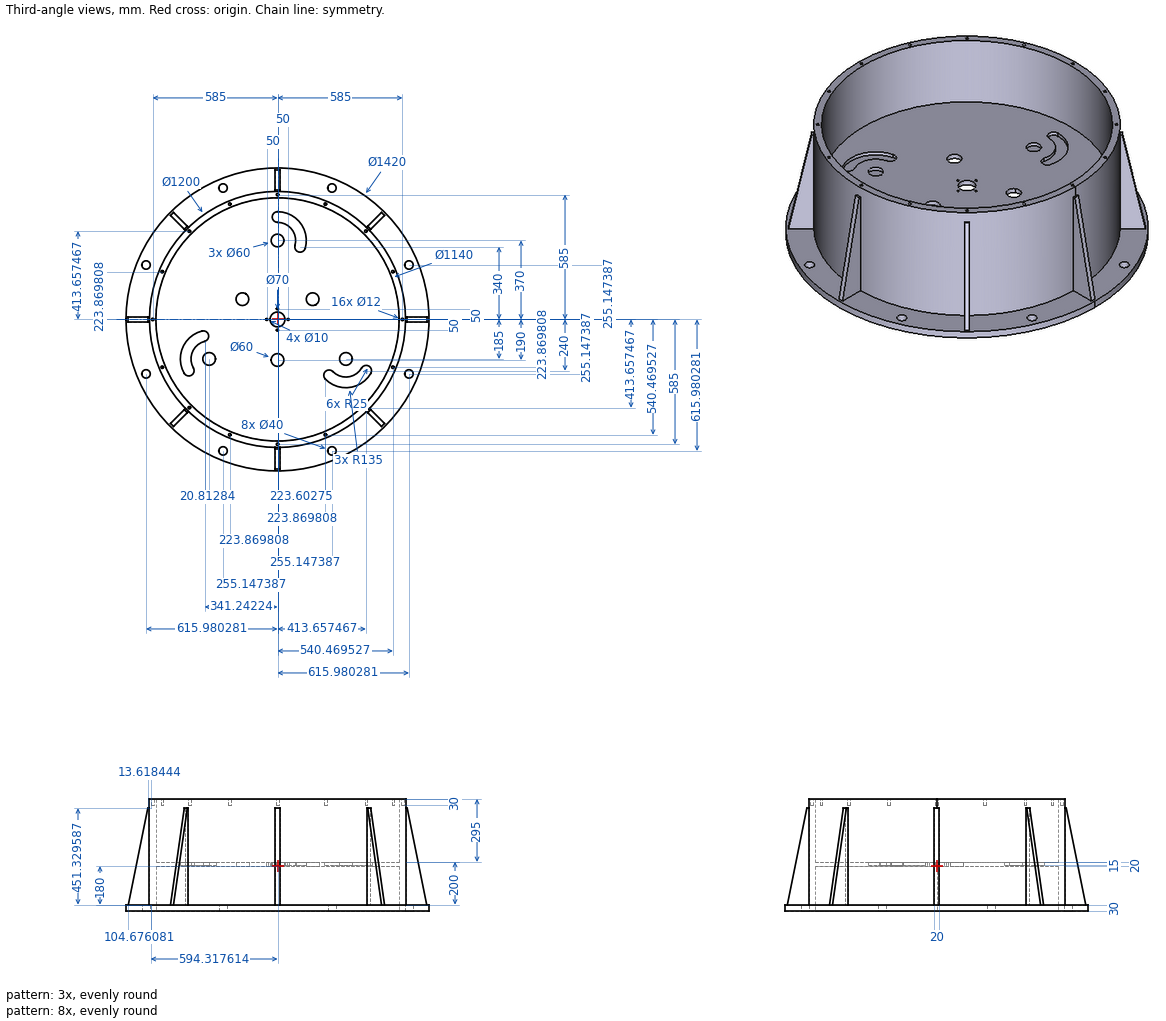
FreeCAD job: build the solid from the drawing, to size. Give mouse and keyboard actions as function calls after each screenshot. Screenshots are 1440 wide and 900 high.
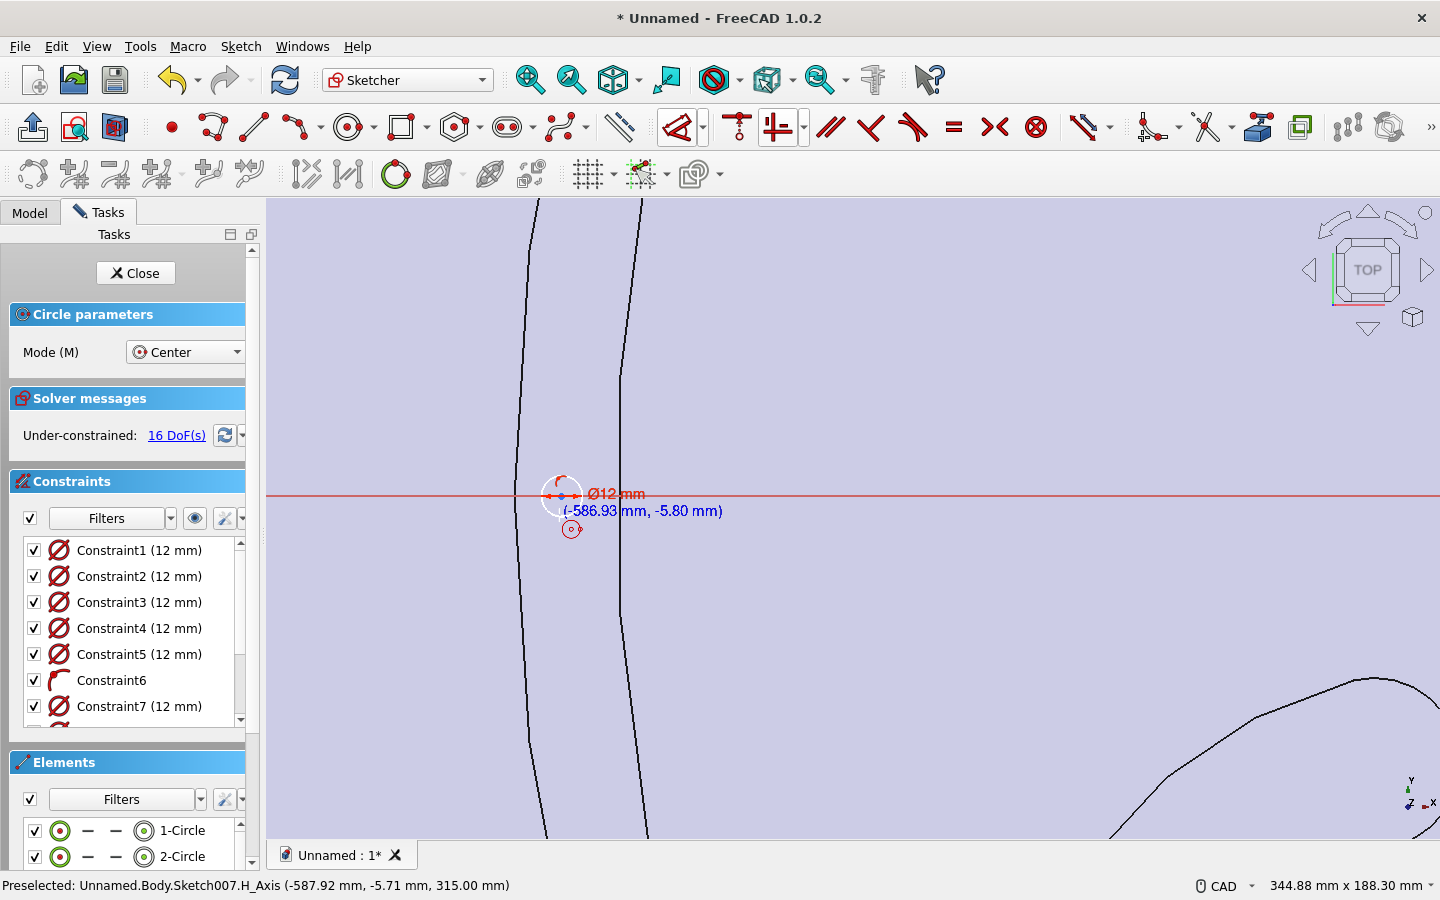
scroll(564, 521, down, 11)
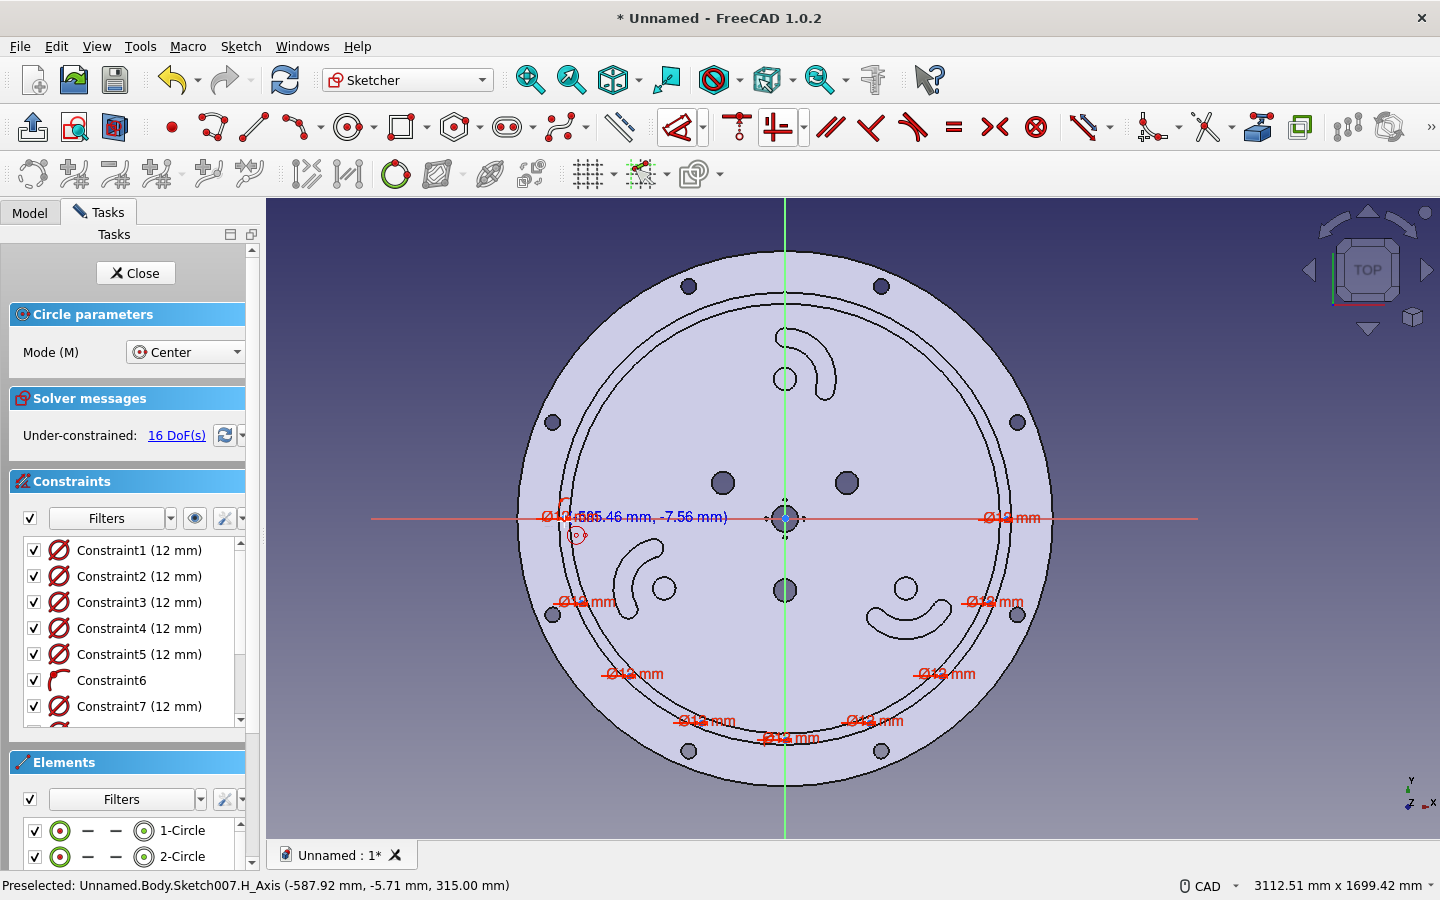
scroll(581, 434, up, 12)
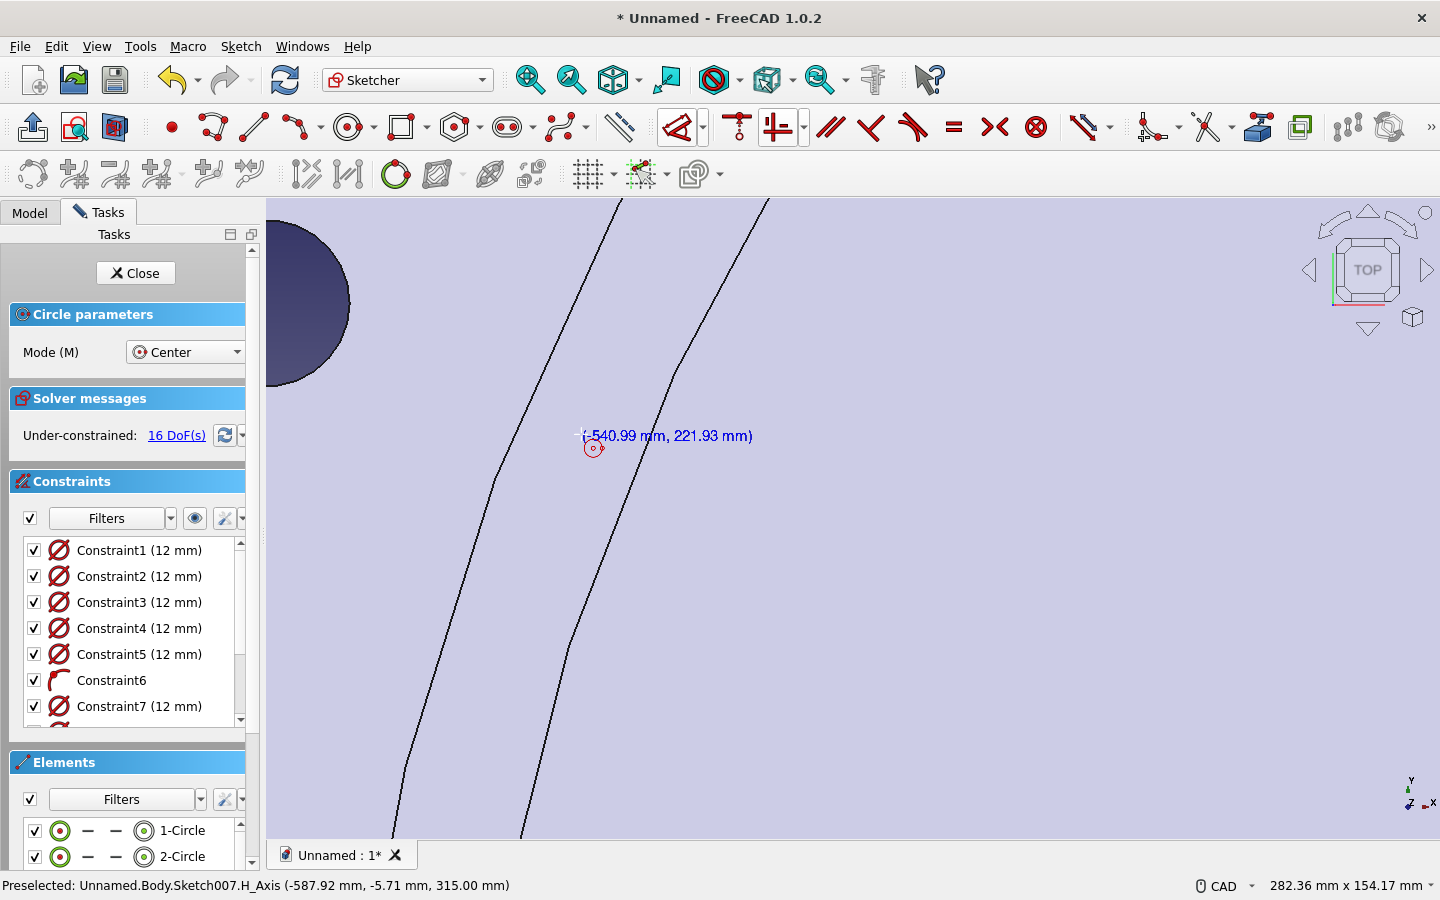
scroll(581, 434, down, 12)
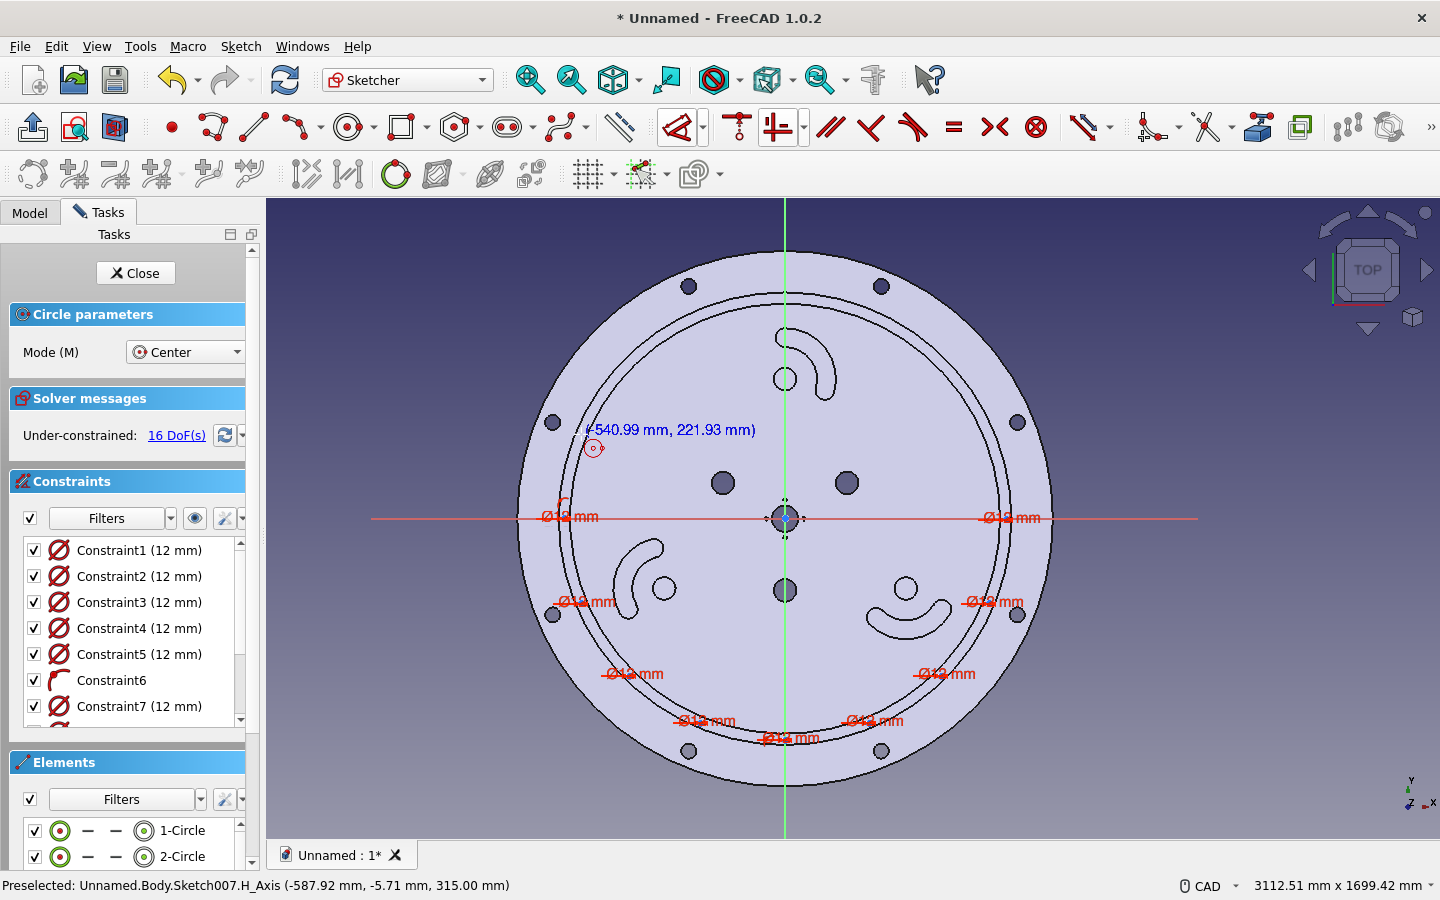
click(581, 434)
move(583, 433)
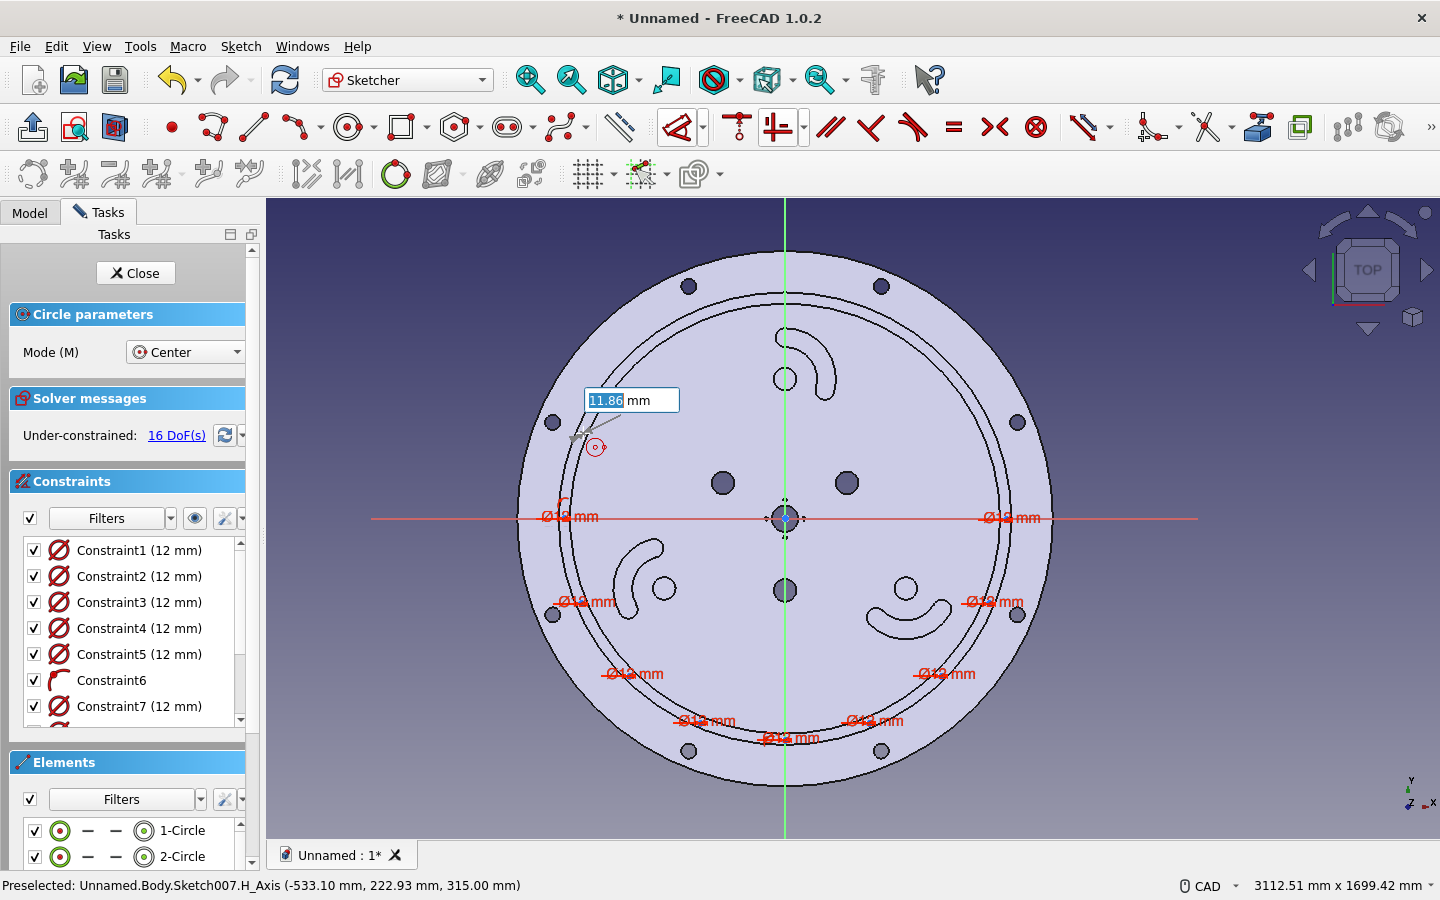
text(12)
key(Return)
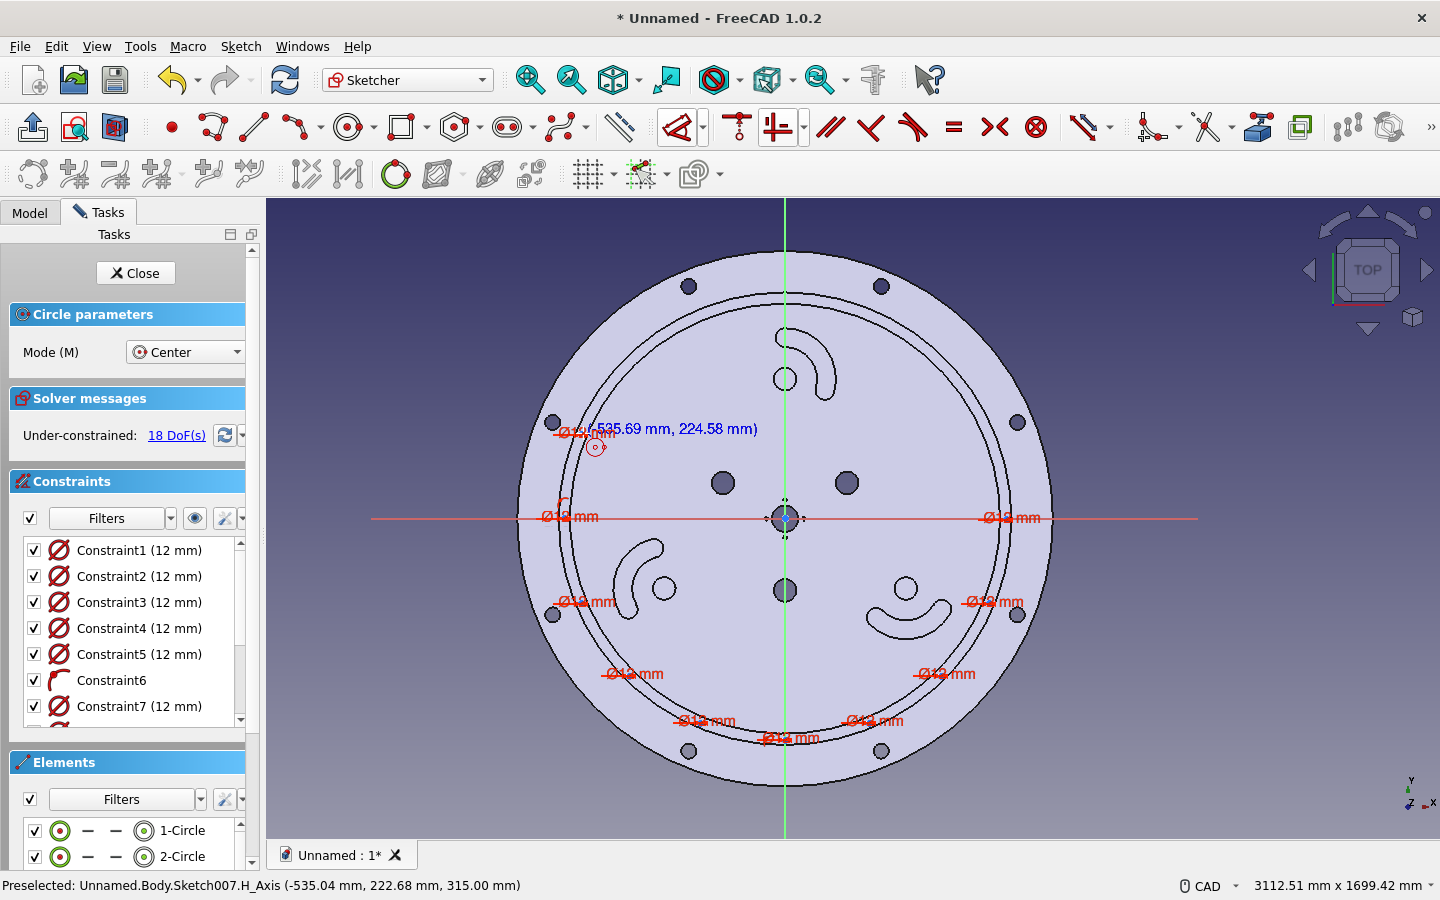
scroll(629, 363, up, 12)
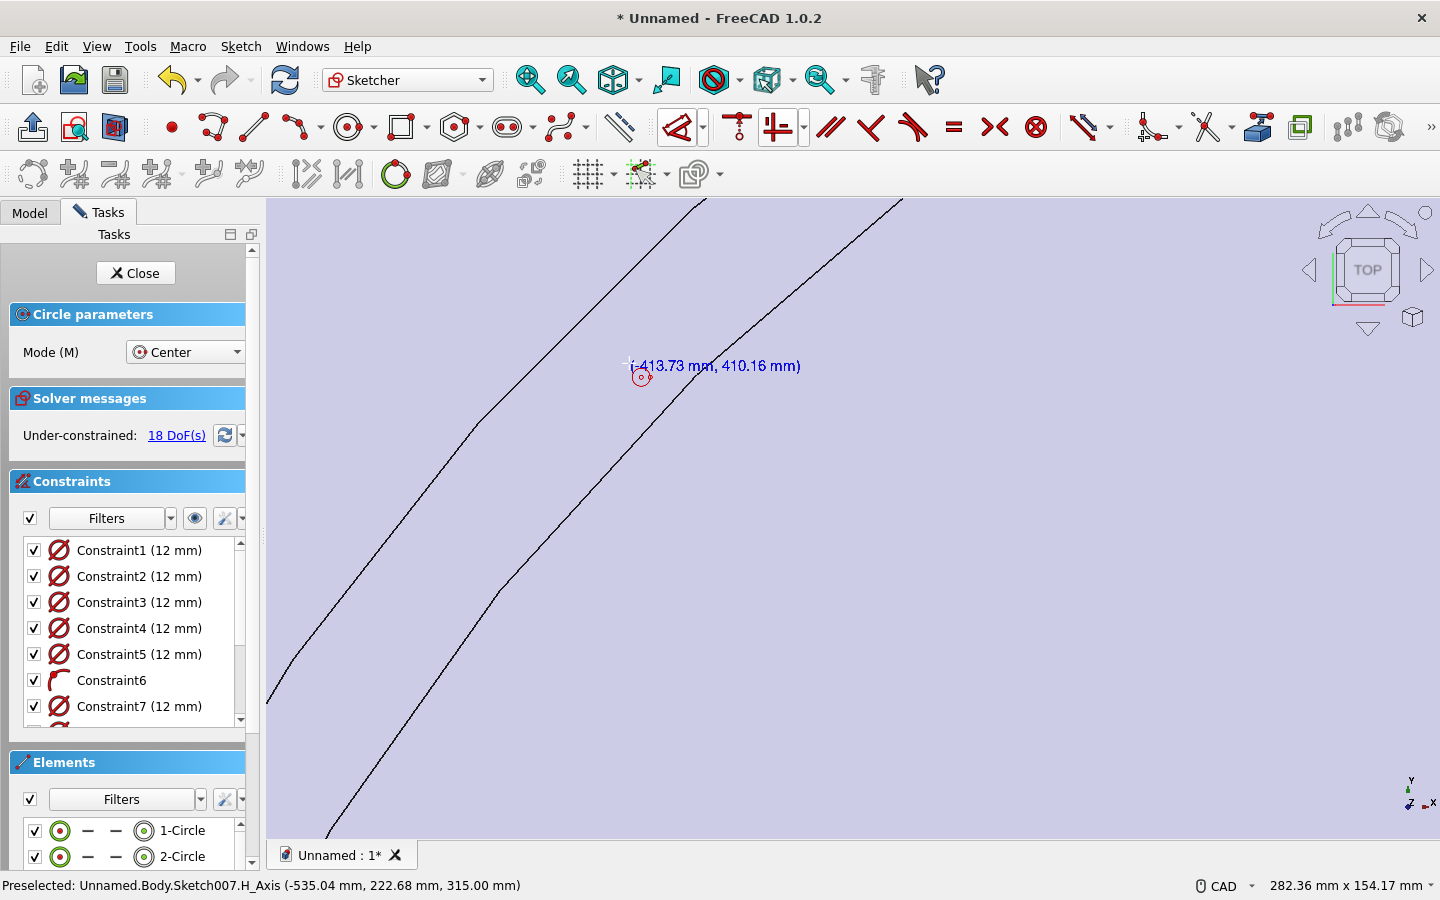
scroll(629, 363, down, 12)